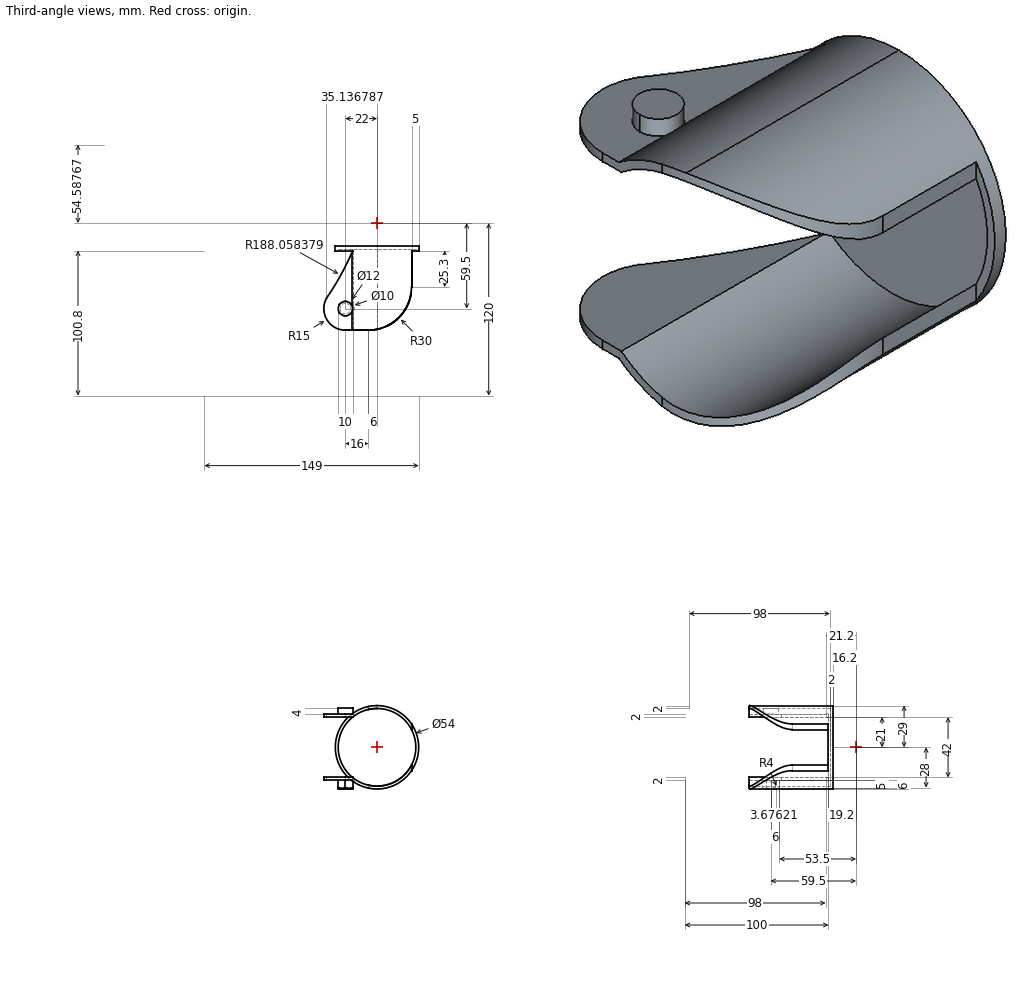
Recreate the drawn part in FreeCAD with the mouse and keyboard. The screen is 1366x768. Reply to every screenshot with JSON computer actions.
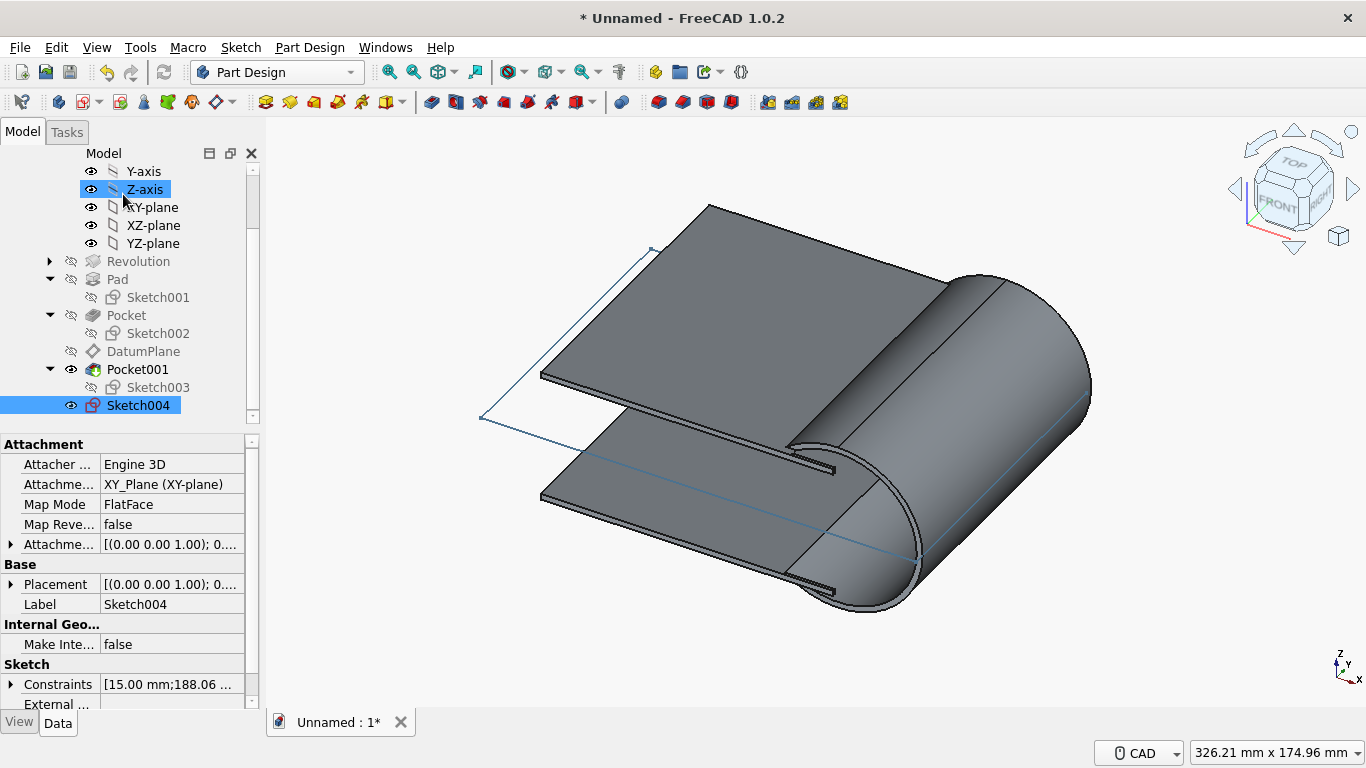
{"action": "left_click", "coordinate": [432, 102]}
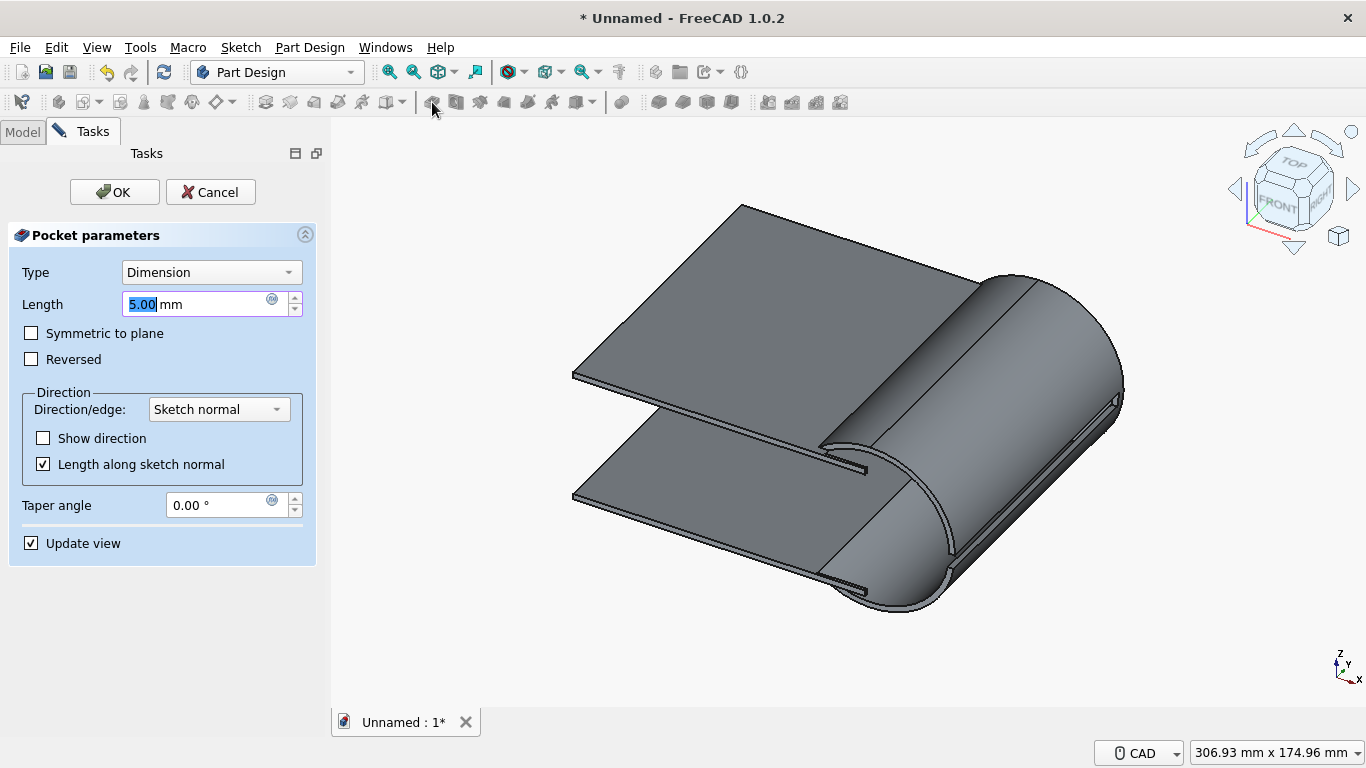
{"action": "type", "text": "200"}
{"action": "key", "text": "Tab"}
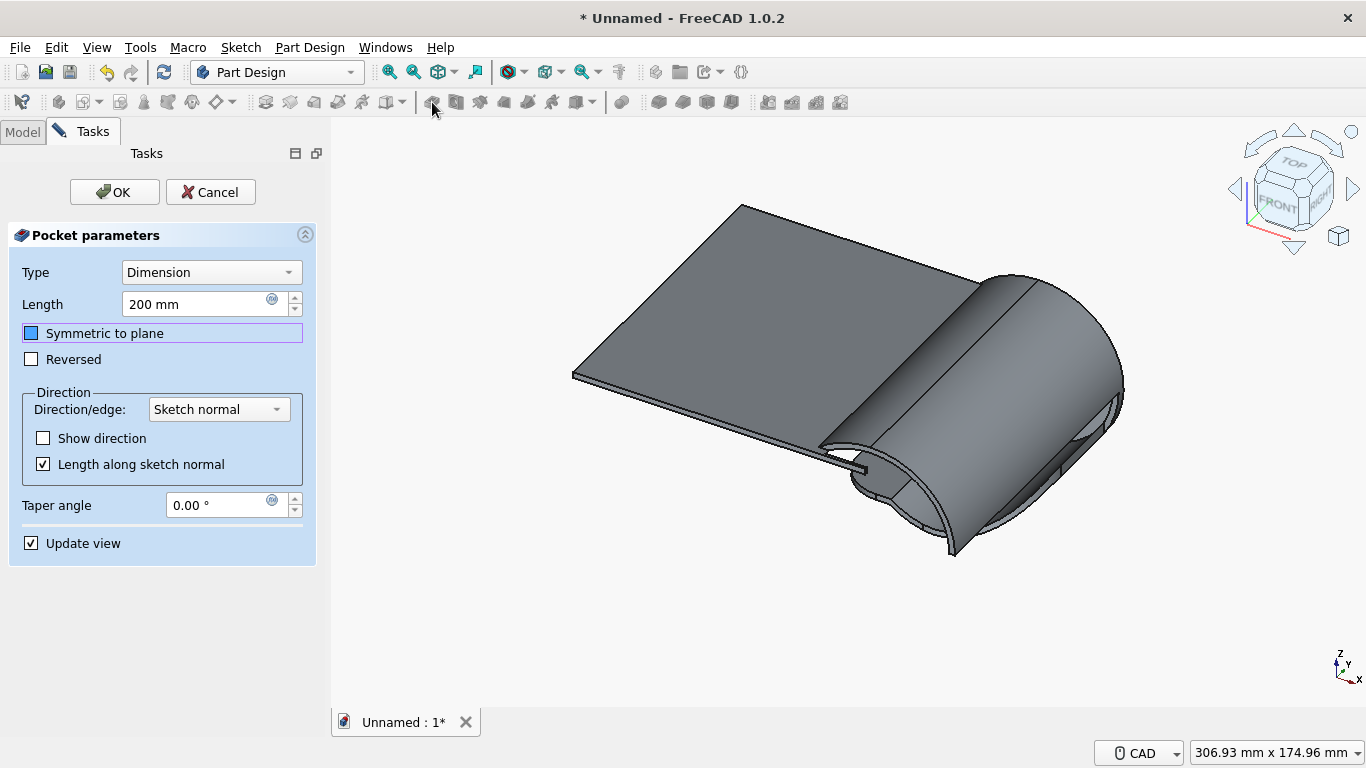
{"action": "left_click", "coordinate": [30, 333]}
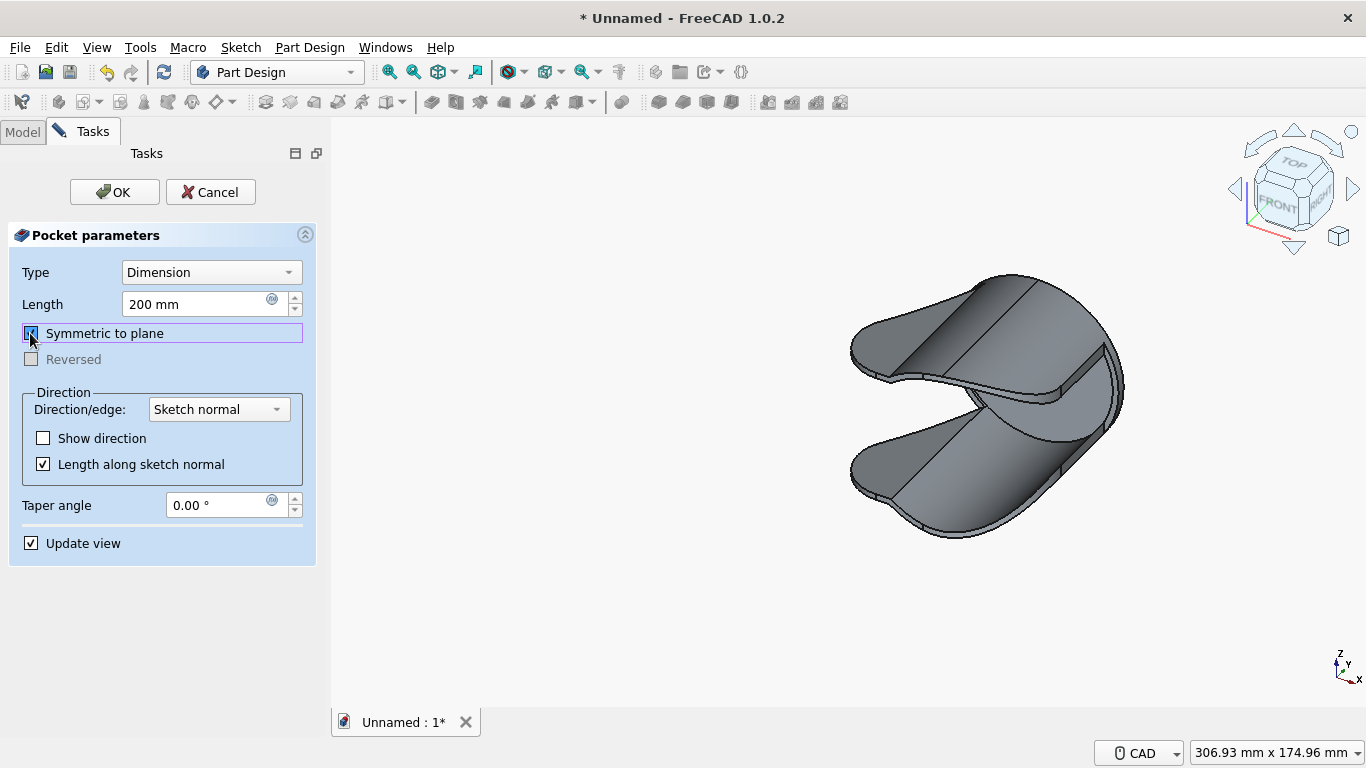
{"action": "left_click", "coordinate": [115, 192]}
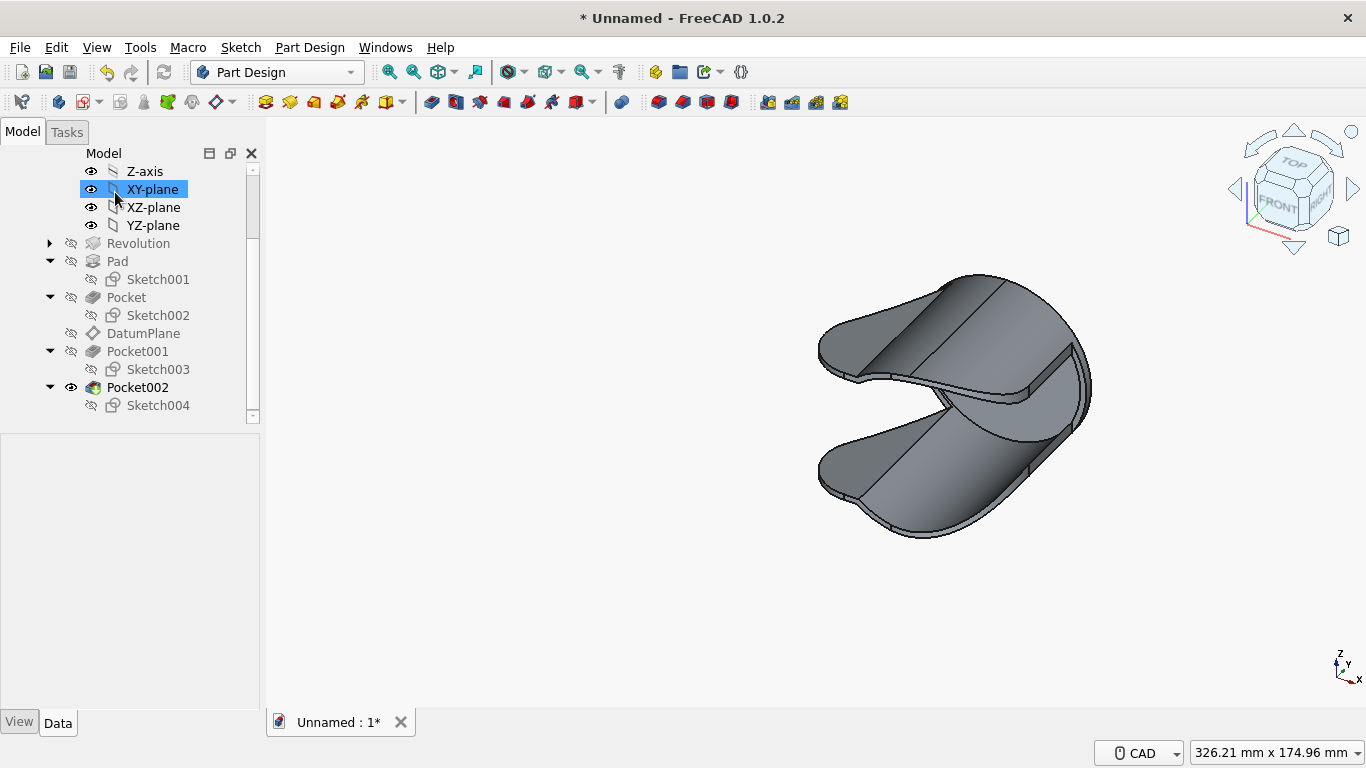
{"action": "left_click", "coordinate": [848, 348]}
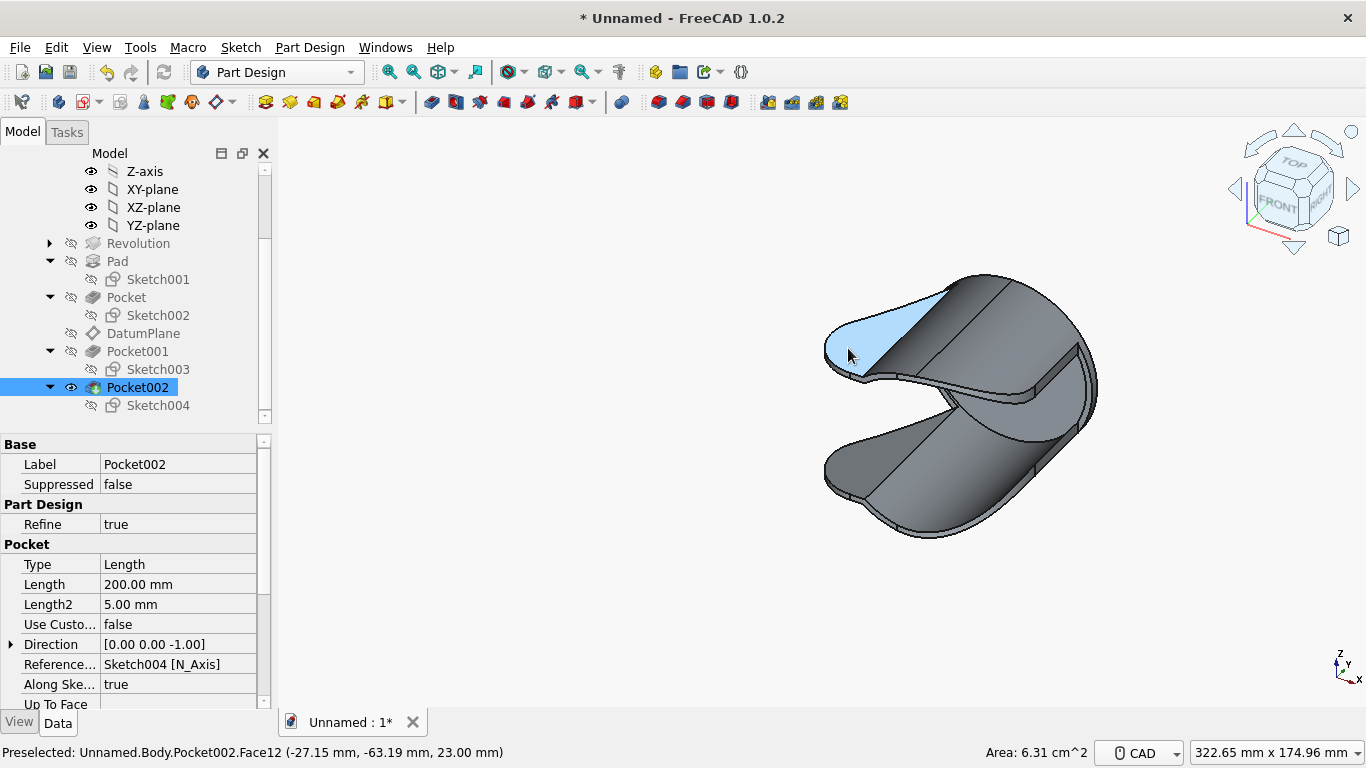
{"action": "left_click", "coordinate": [84, 102]}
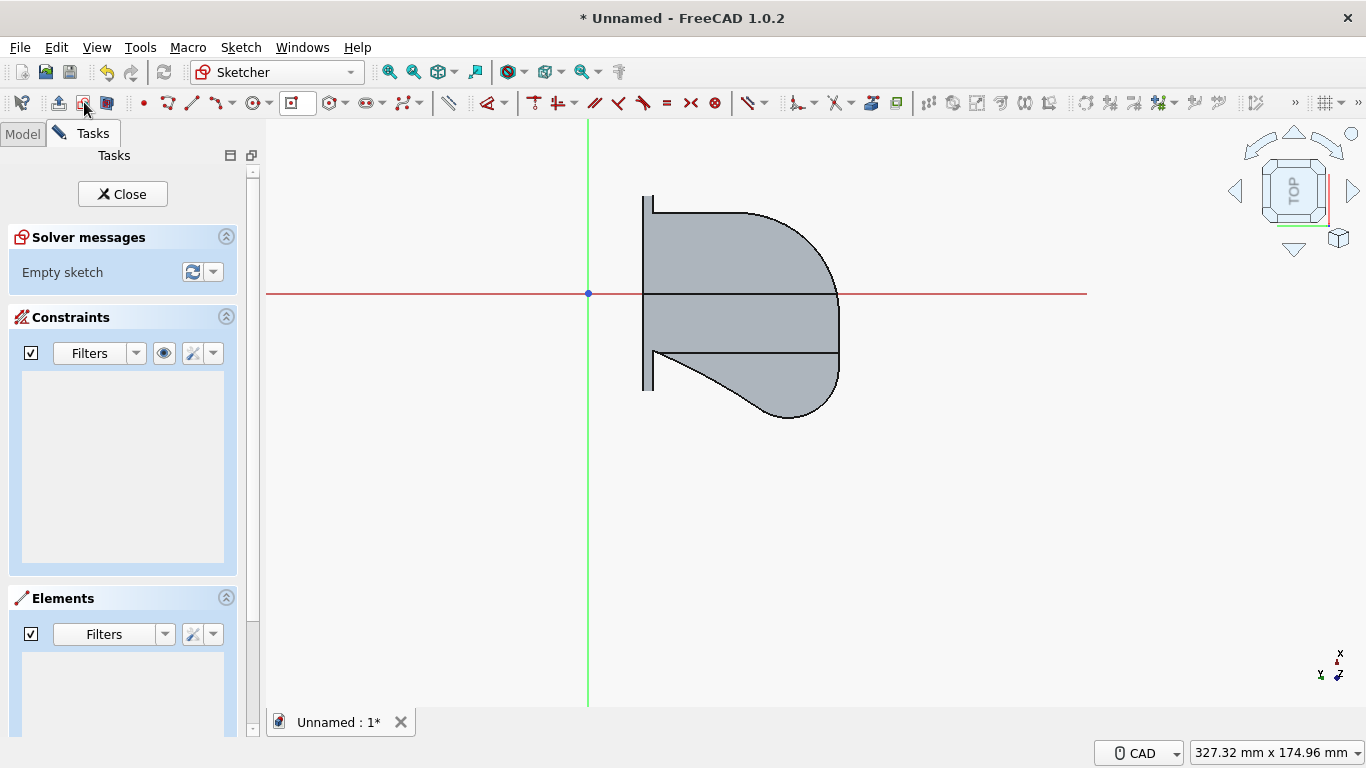
{"action": "left_click", "coordinate": [108, 104]}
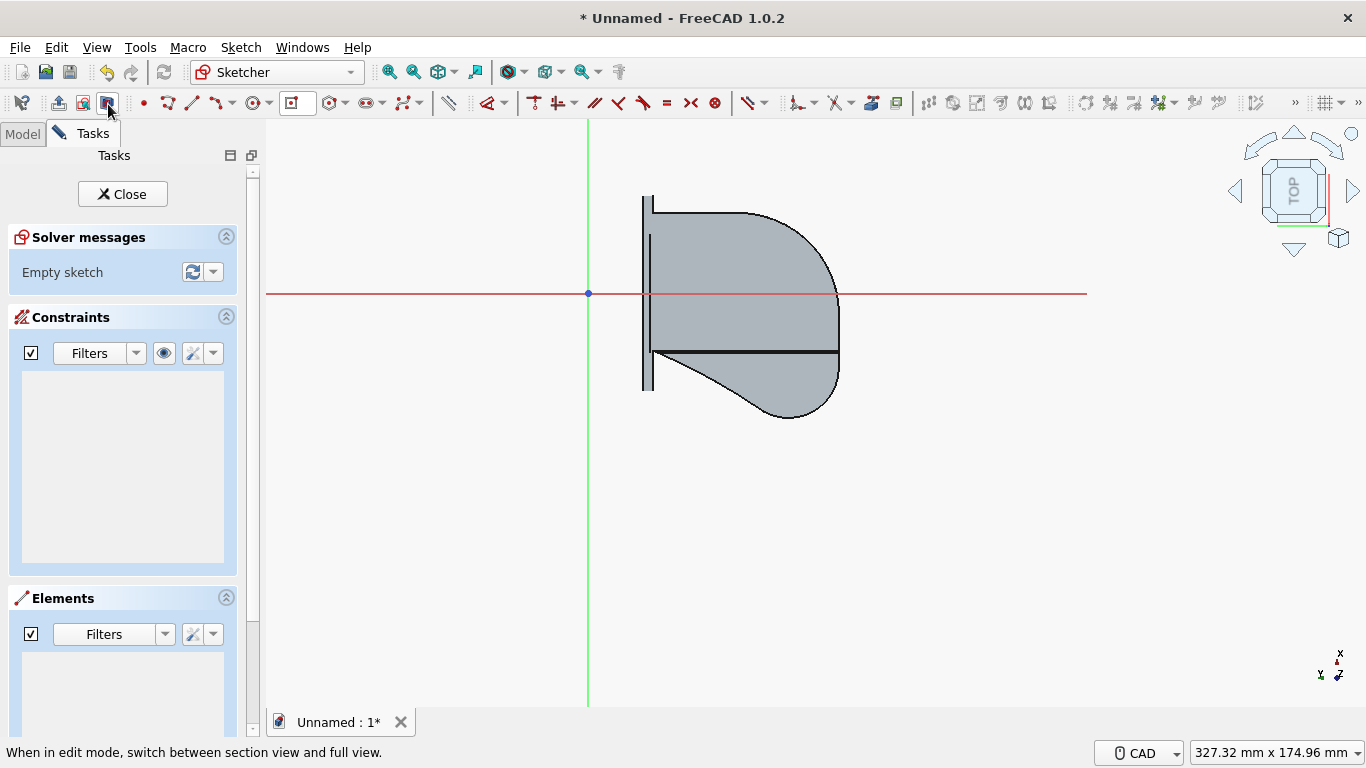
{"action": "scroll", "coordinate": [793, 363], "scroll_direction": "up", "scroll_amount": 12}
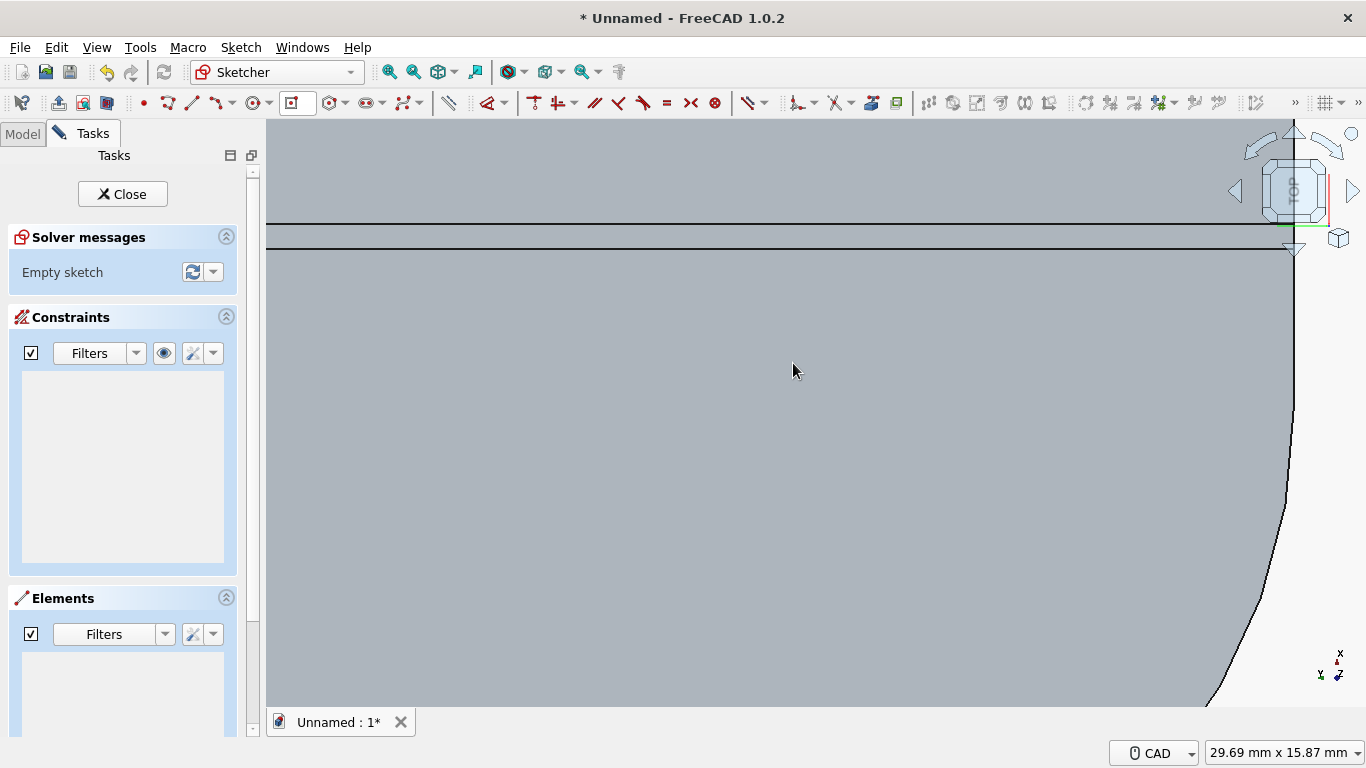
{"action": "left_click", "coordinate": [254, 104]}